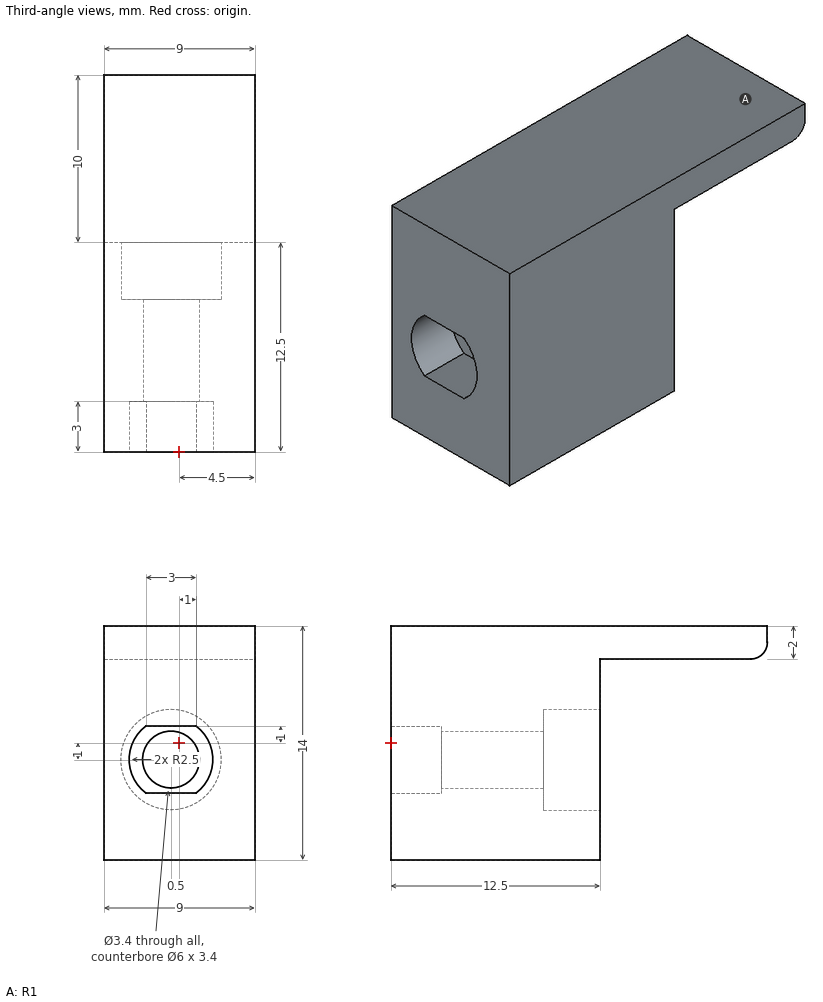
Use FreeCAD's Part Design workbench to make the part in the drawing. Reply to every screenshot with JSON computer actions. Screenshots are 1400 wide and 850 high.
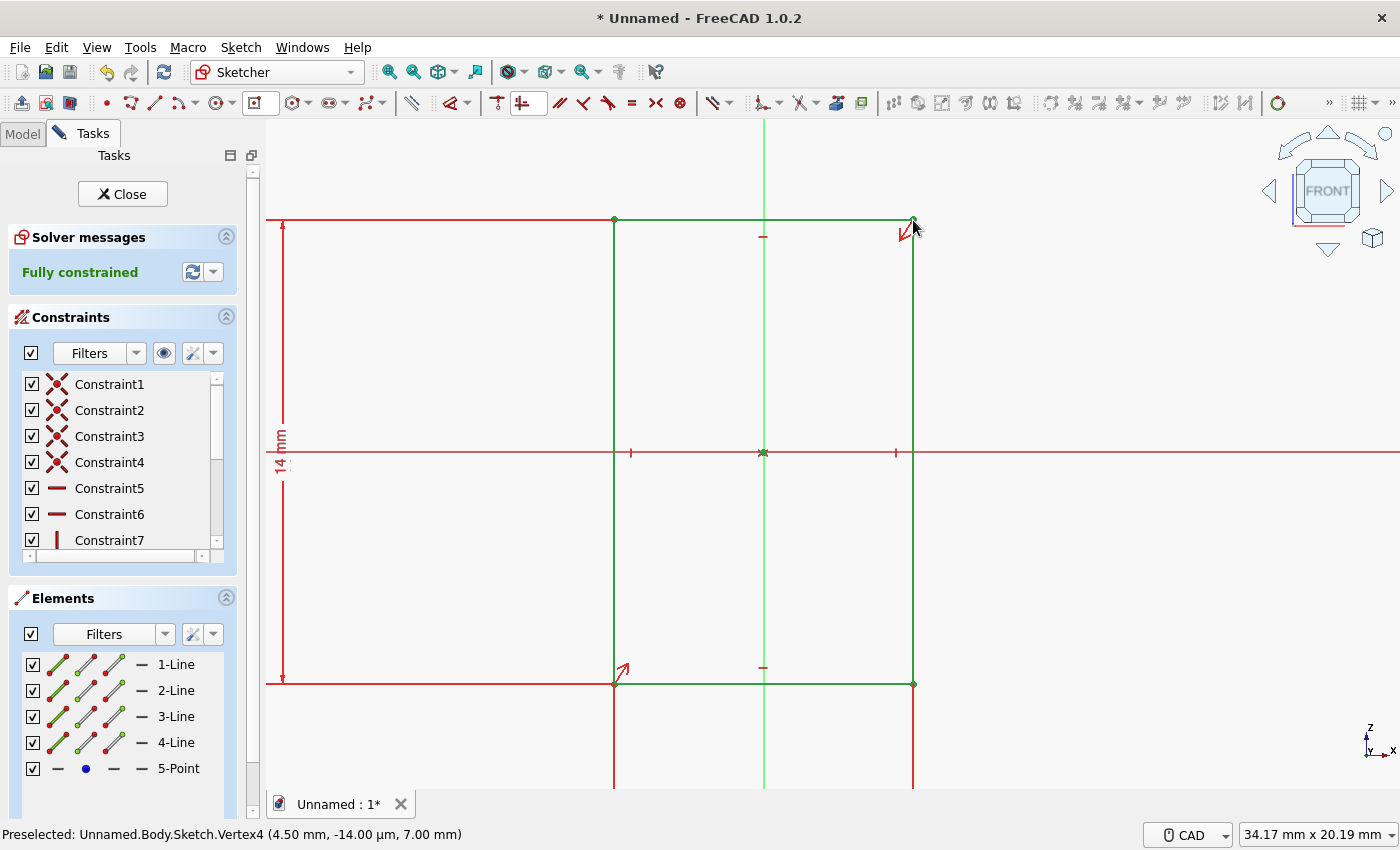
{"action": "left_click", "coordinate": [123, 194]}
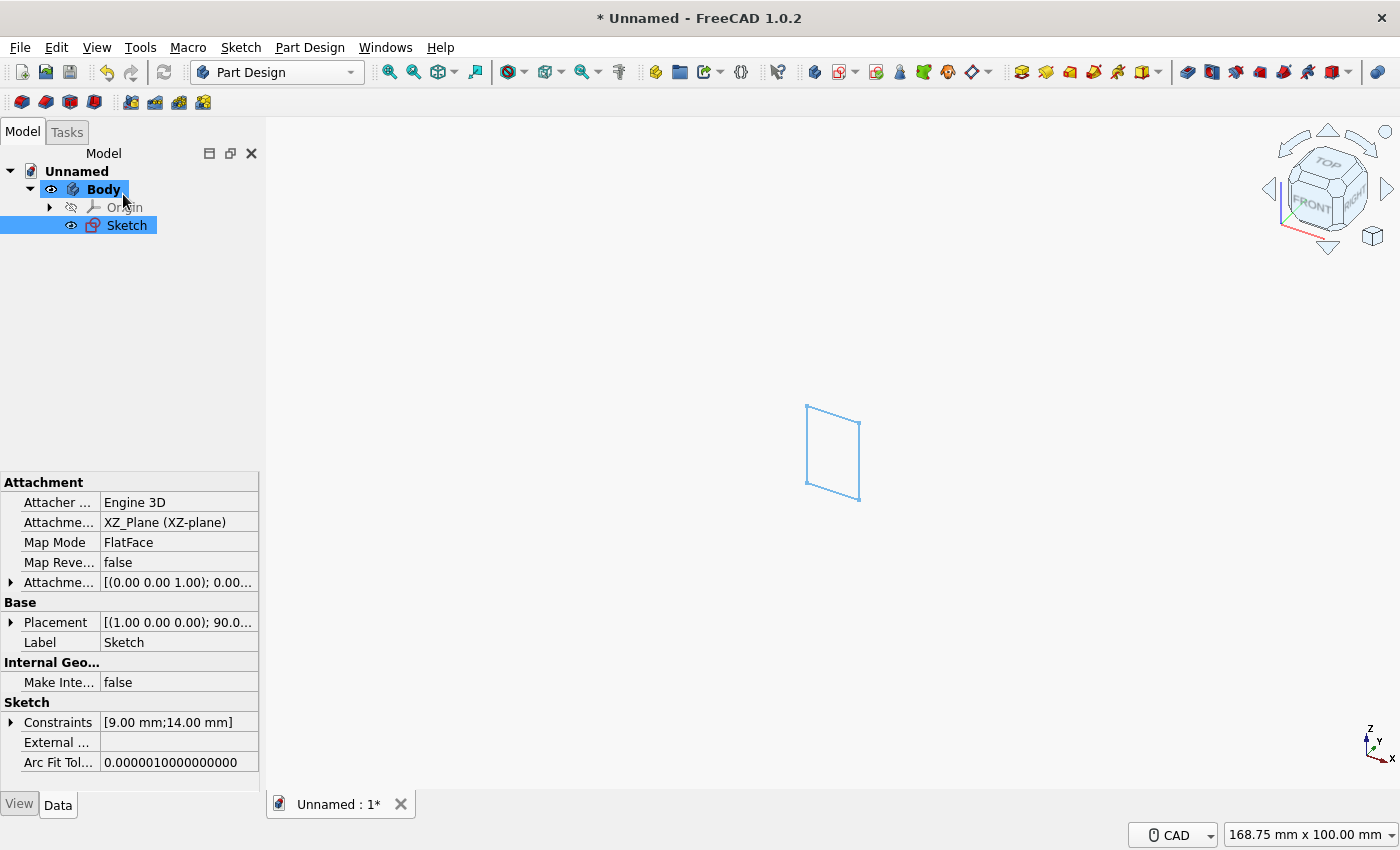
{"action": "left_click", "coordinate": [1022, 72]}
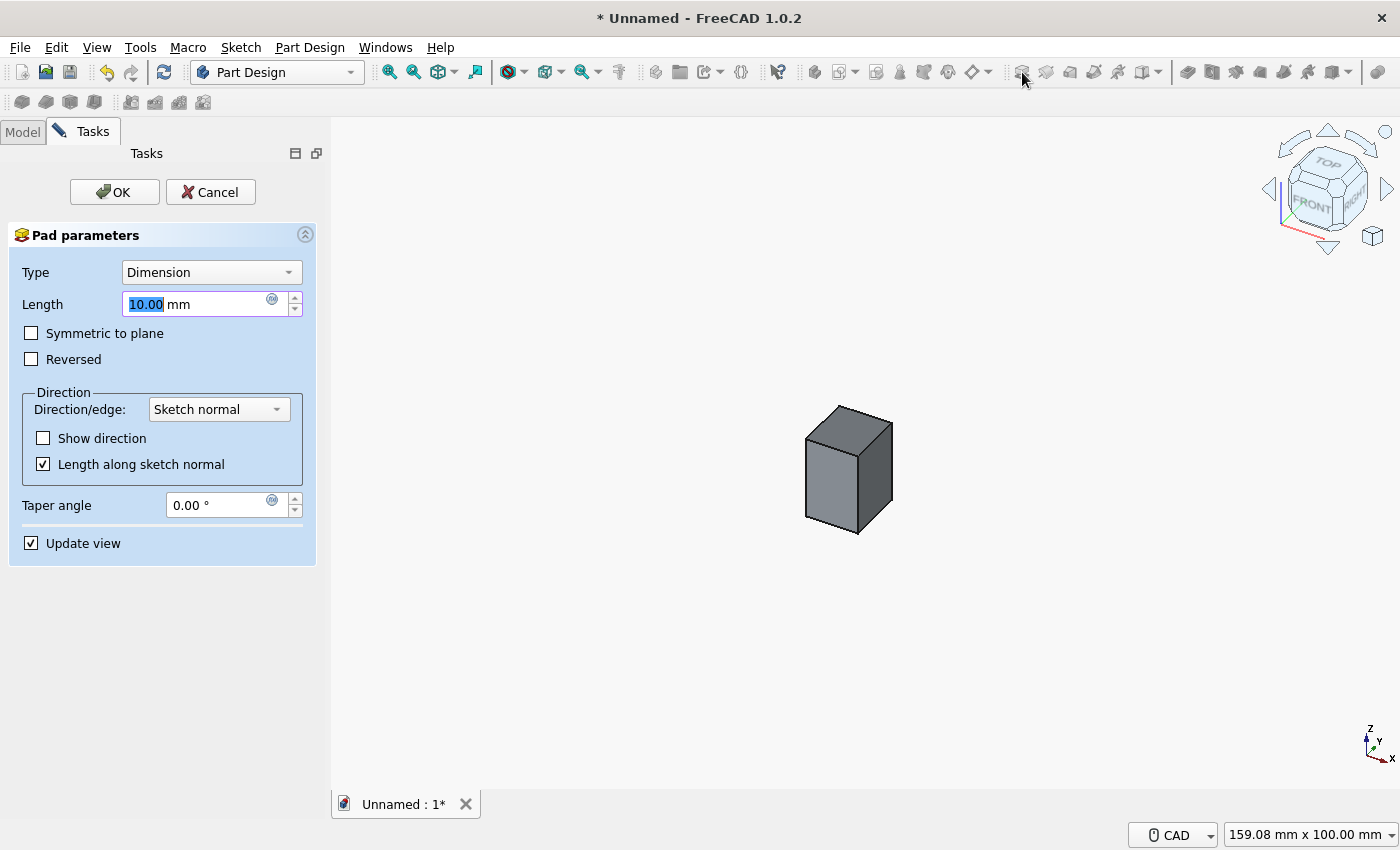
{"action": "type", "text": "12.5"}
{"action": "key", "text": "Tab"}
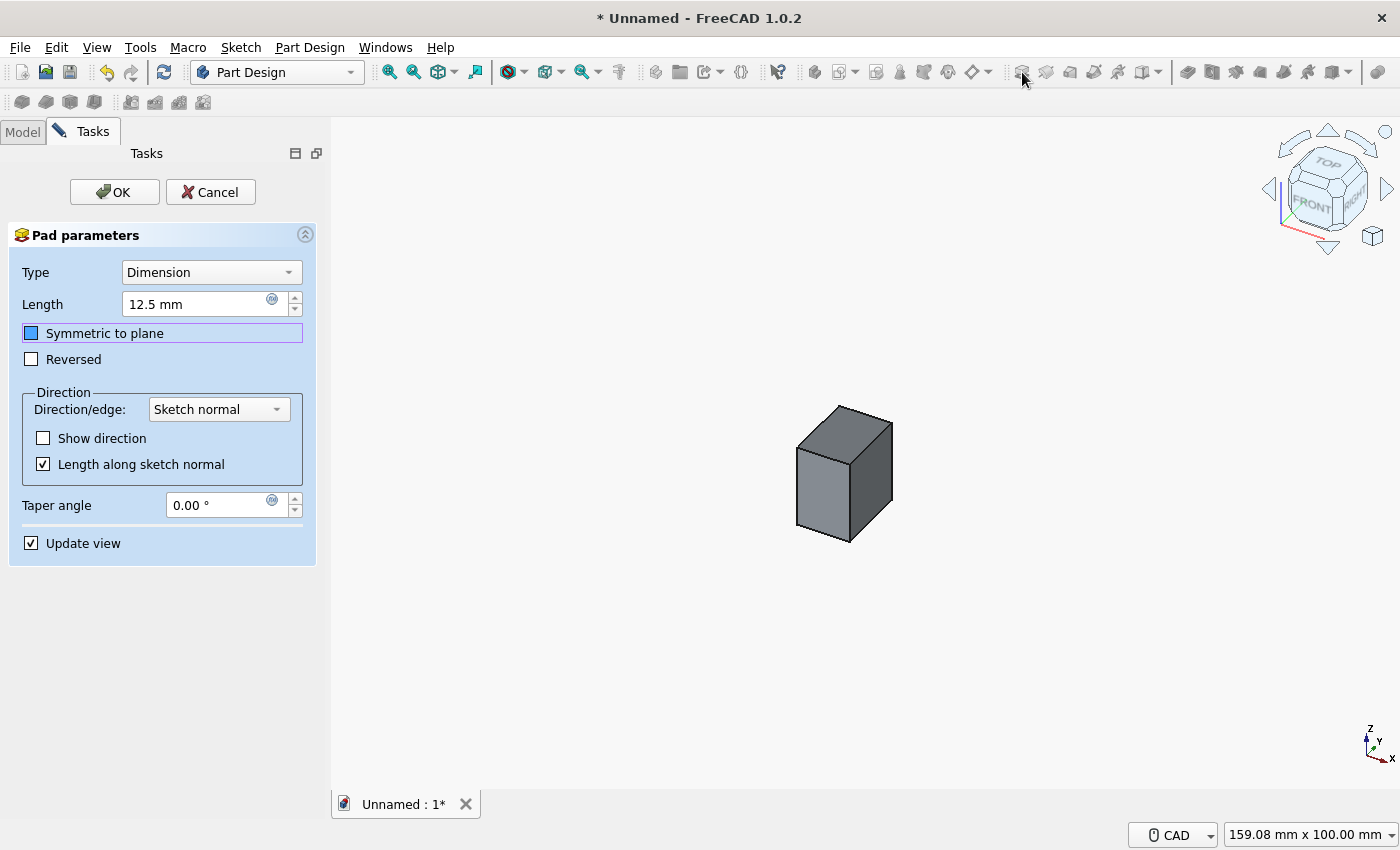
{"action": "left_click", "coordinate": [30, 359]}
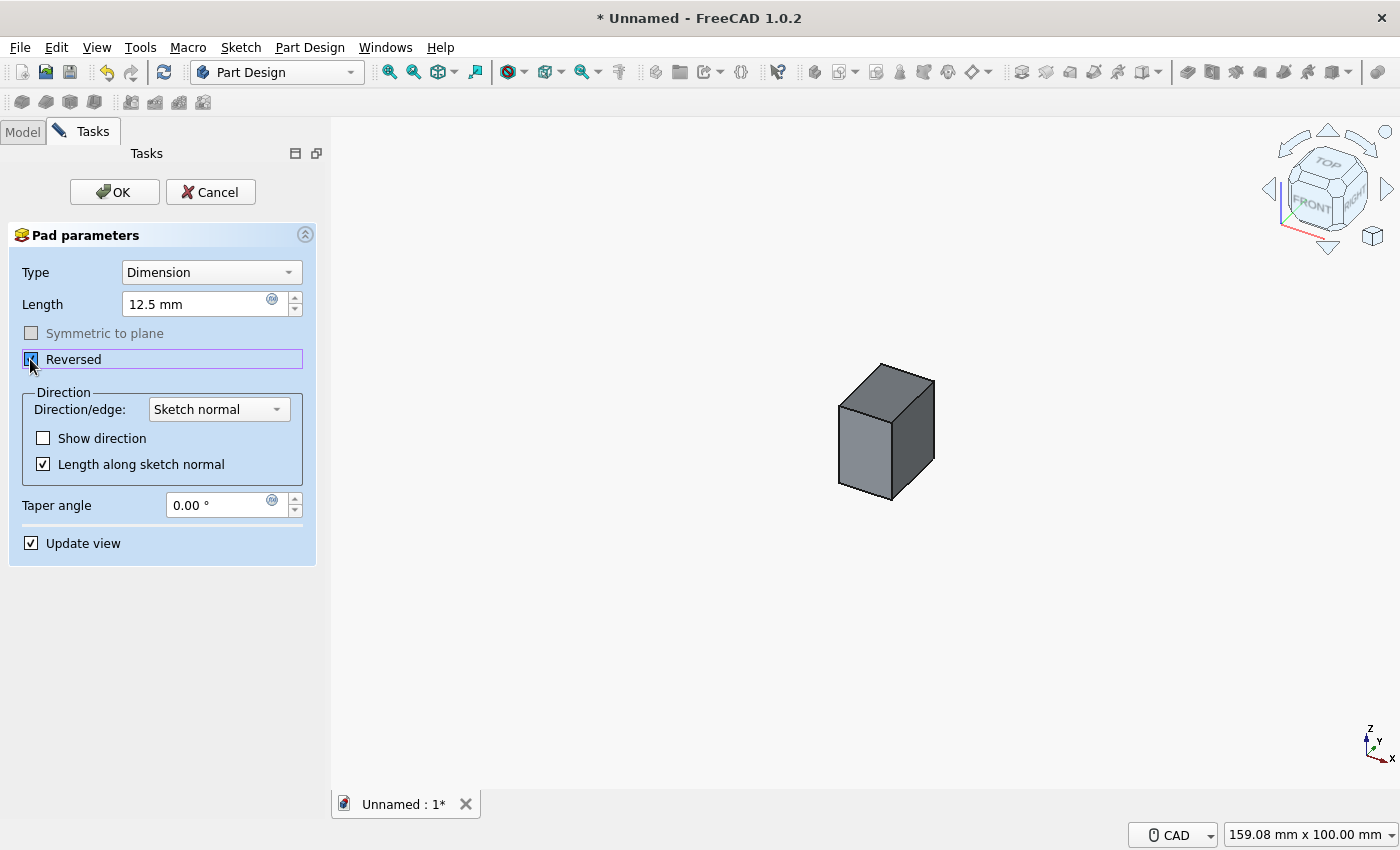
{"action": "left_click", "coordinate": [115, 192]}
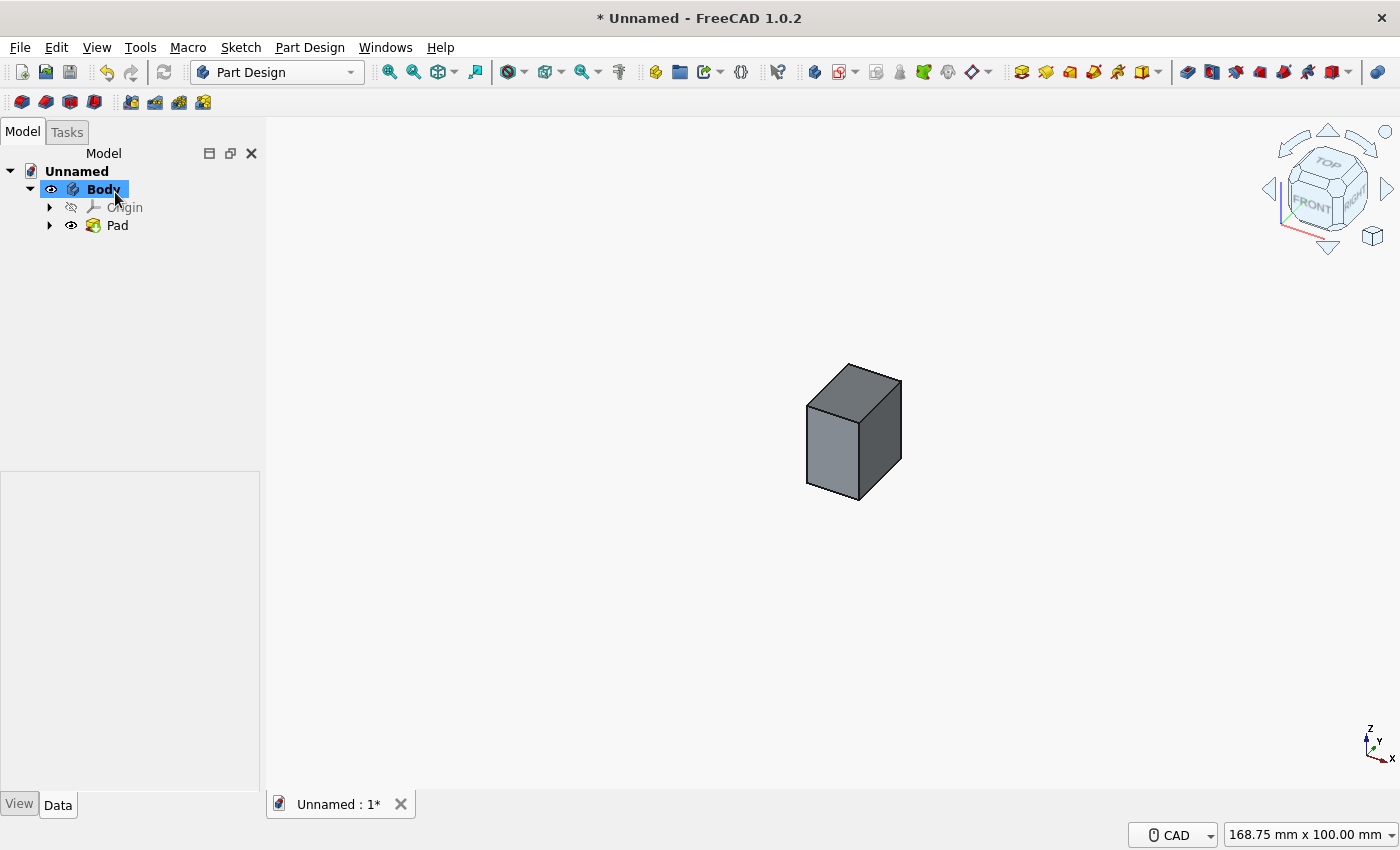
{"action": "key", "text": "v f"}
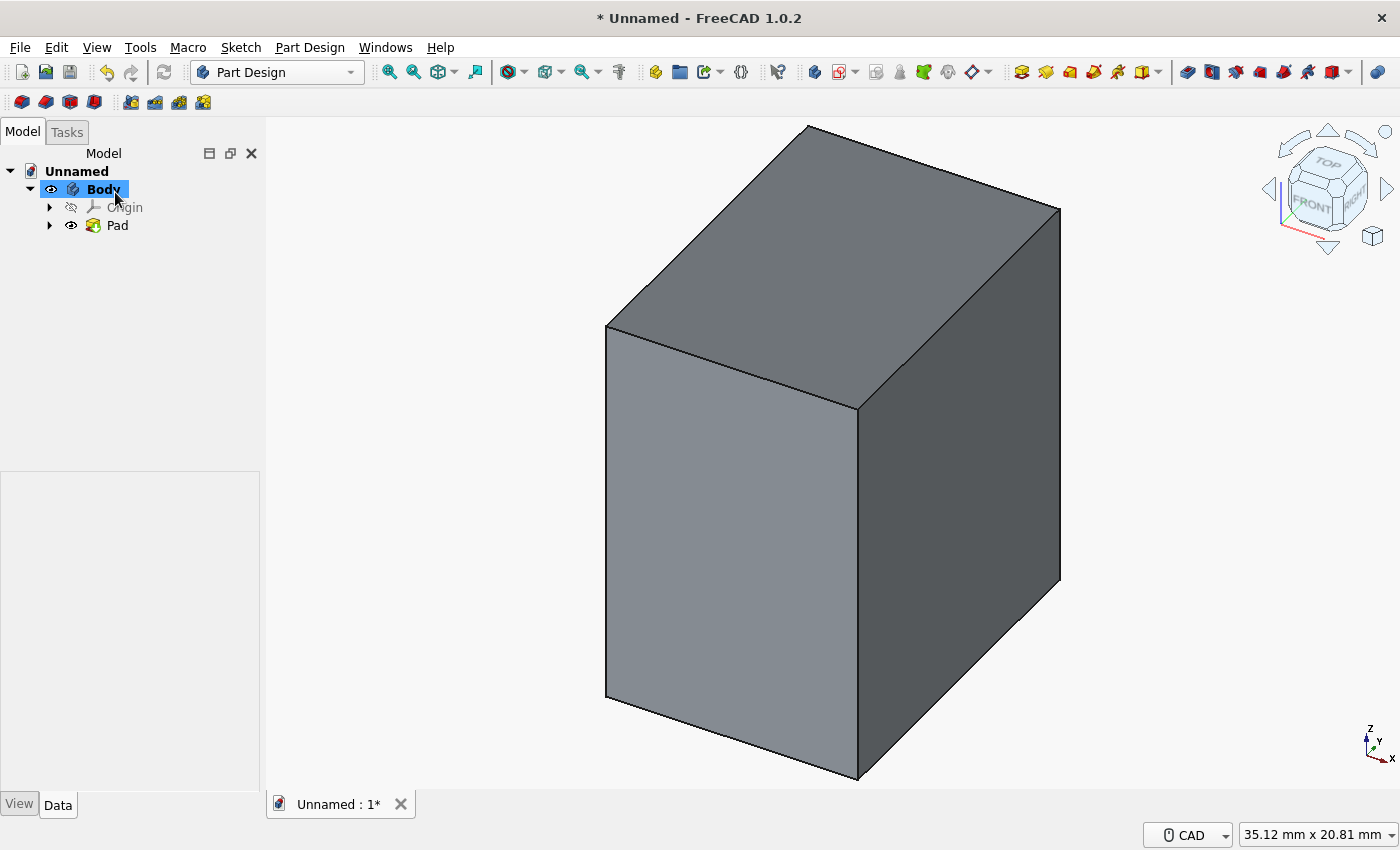
{"action": "left_click", "coordinate": [840, 72]}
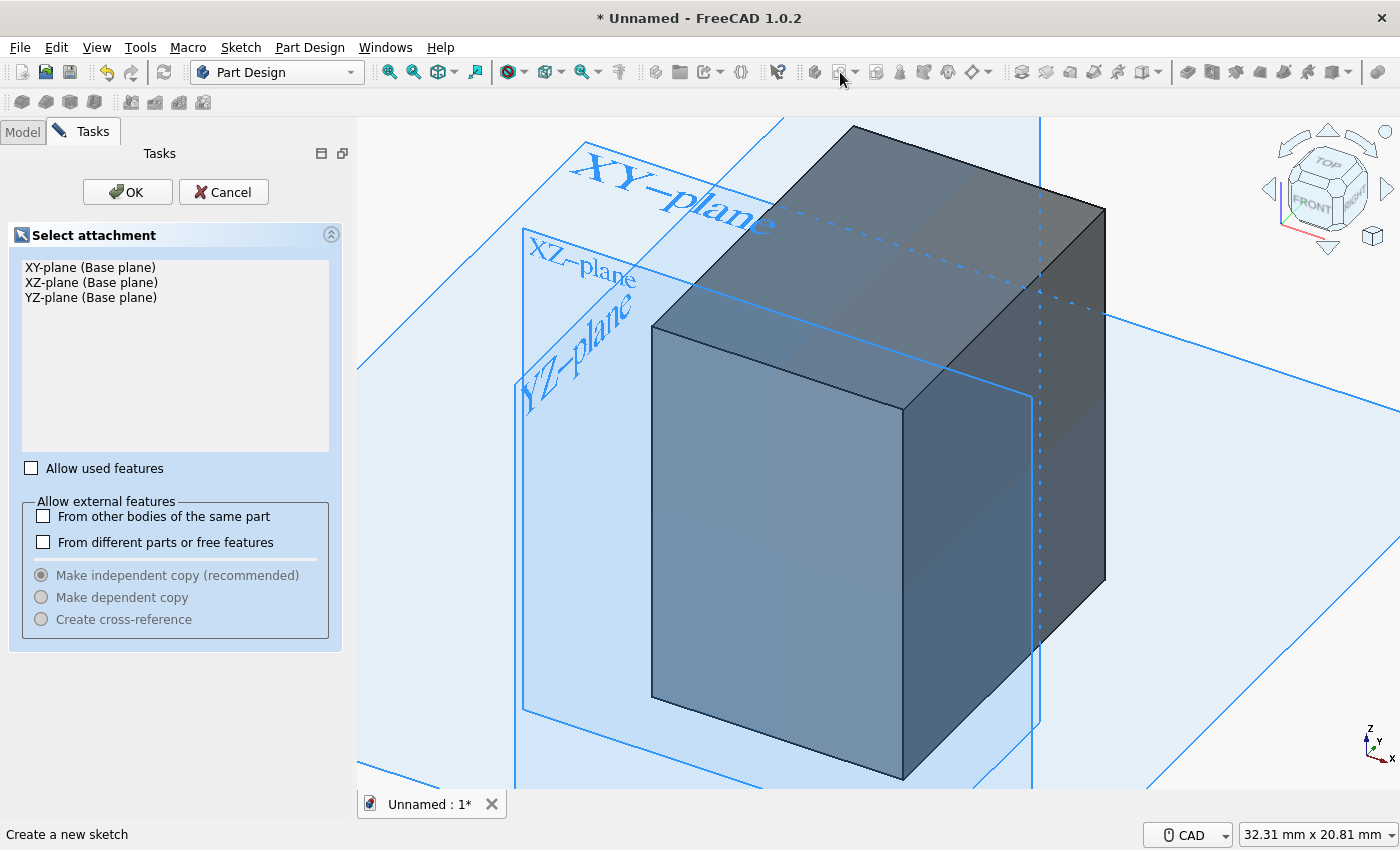
{"action": "left_click", "coordinate": [82, 282]}